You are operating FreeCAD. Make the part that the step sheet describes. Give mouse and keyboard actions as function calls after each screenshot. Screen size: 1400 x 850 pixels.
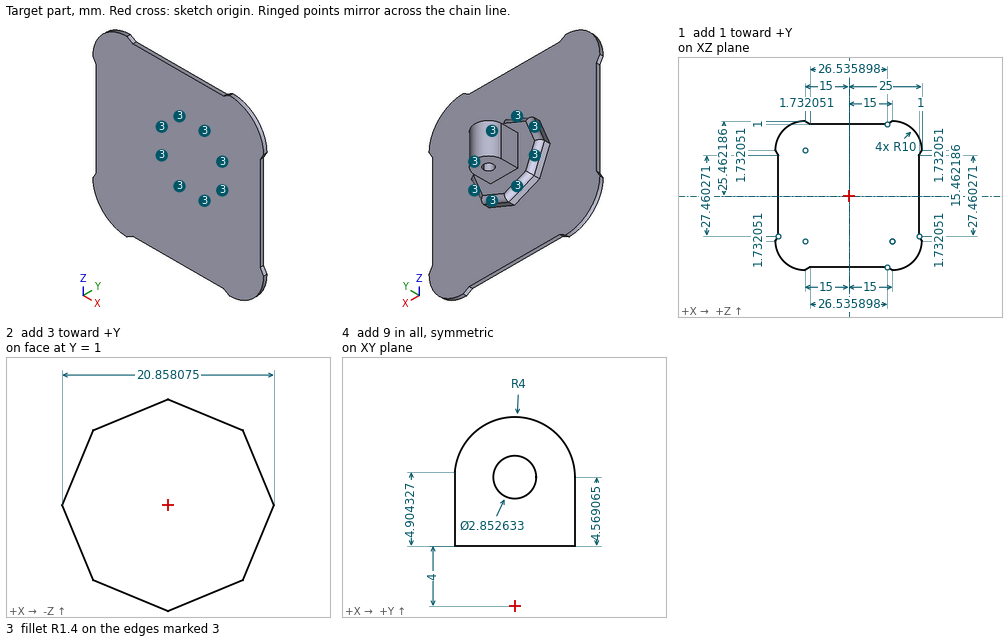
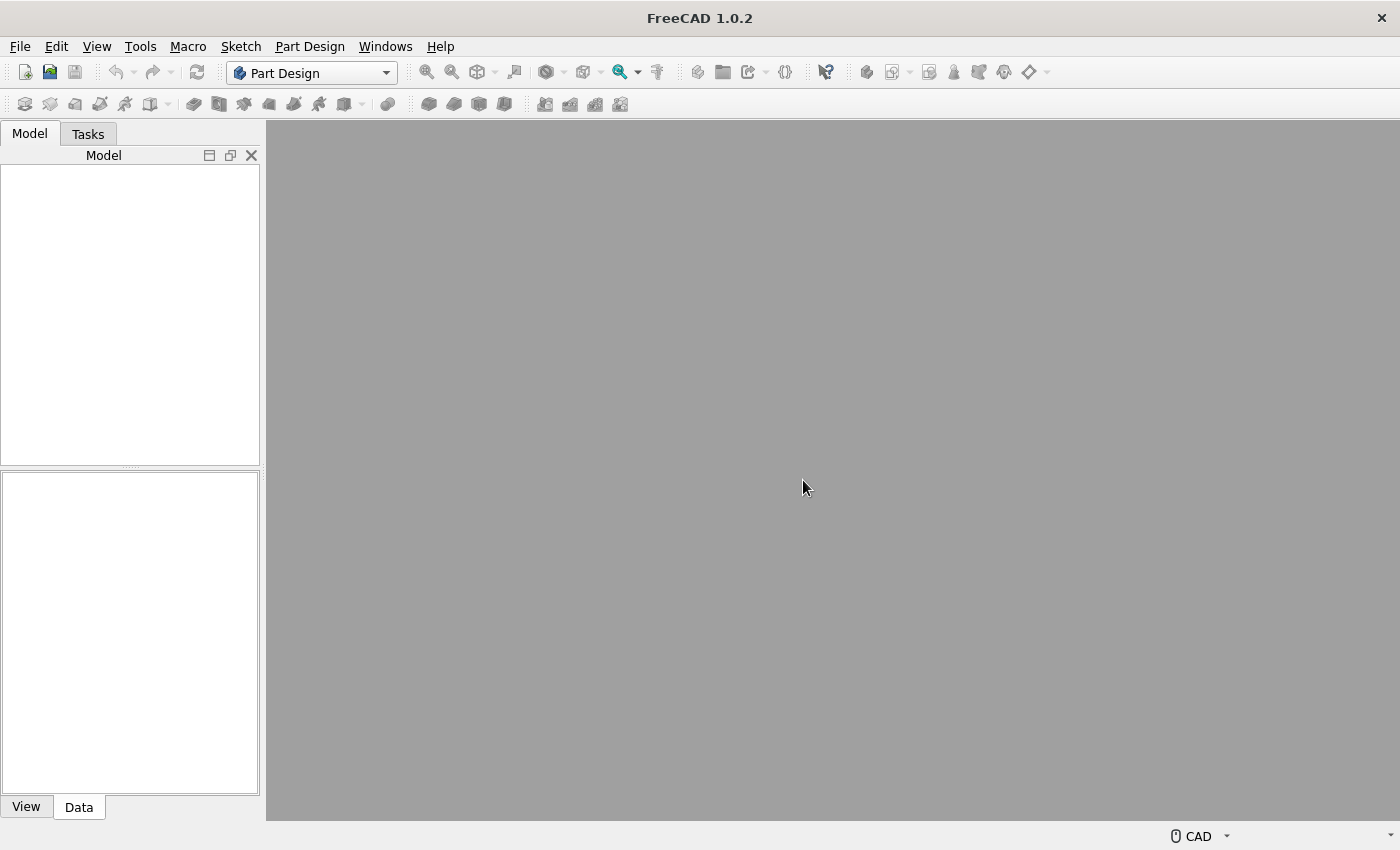
click(25, 72)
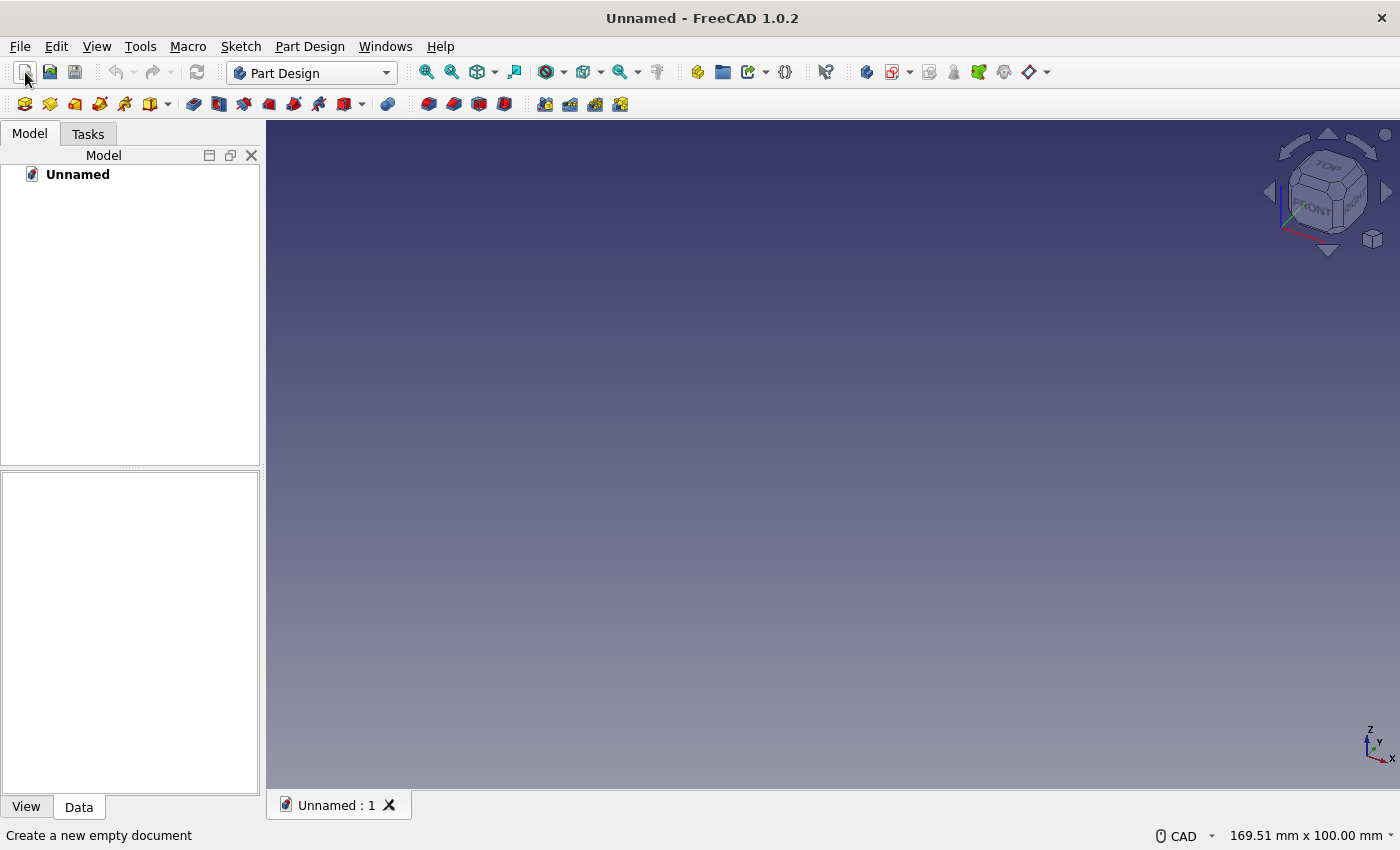
click(892, 72)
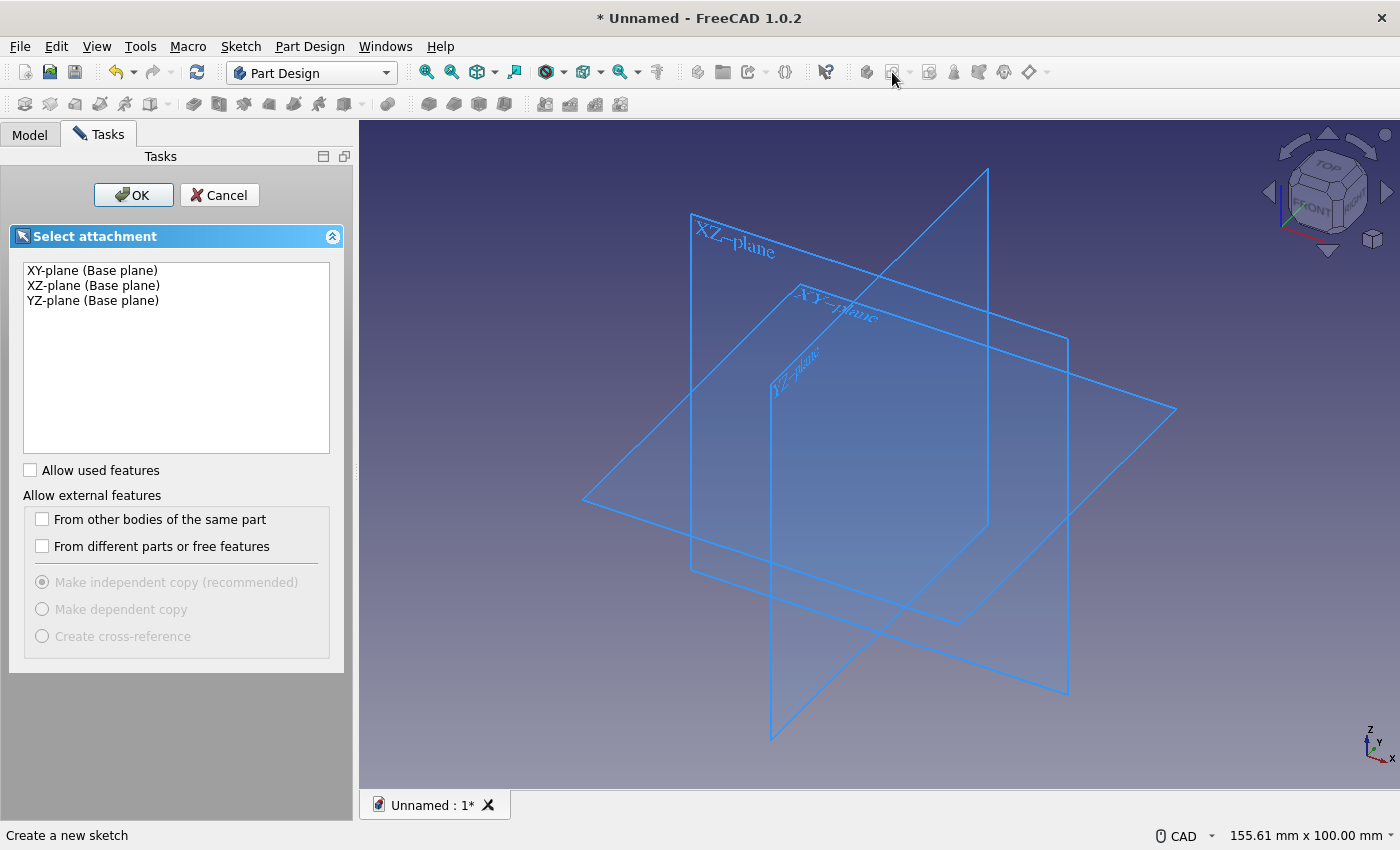
click(84, 286)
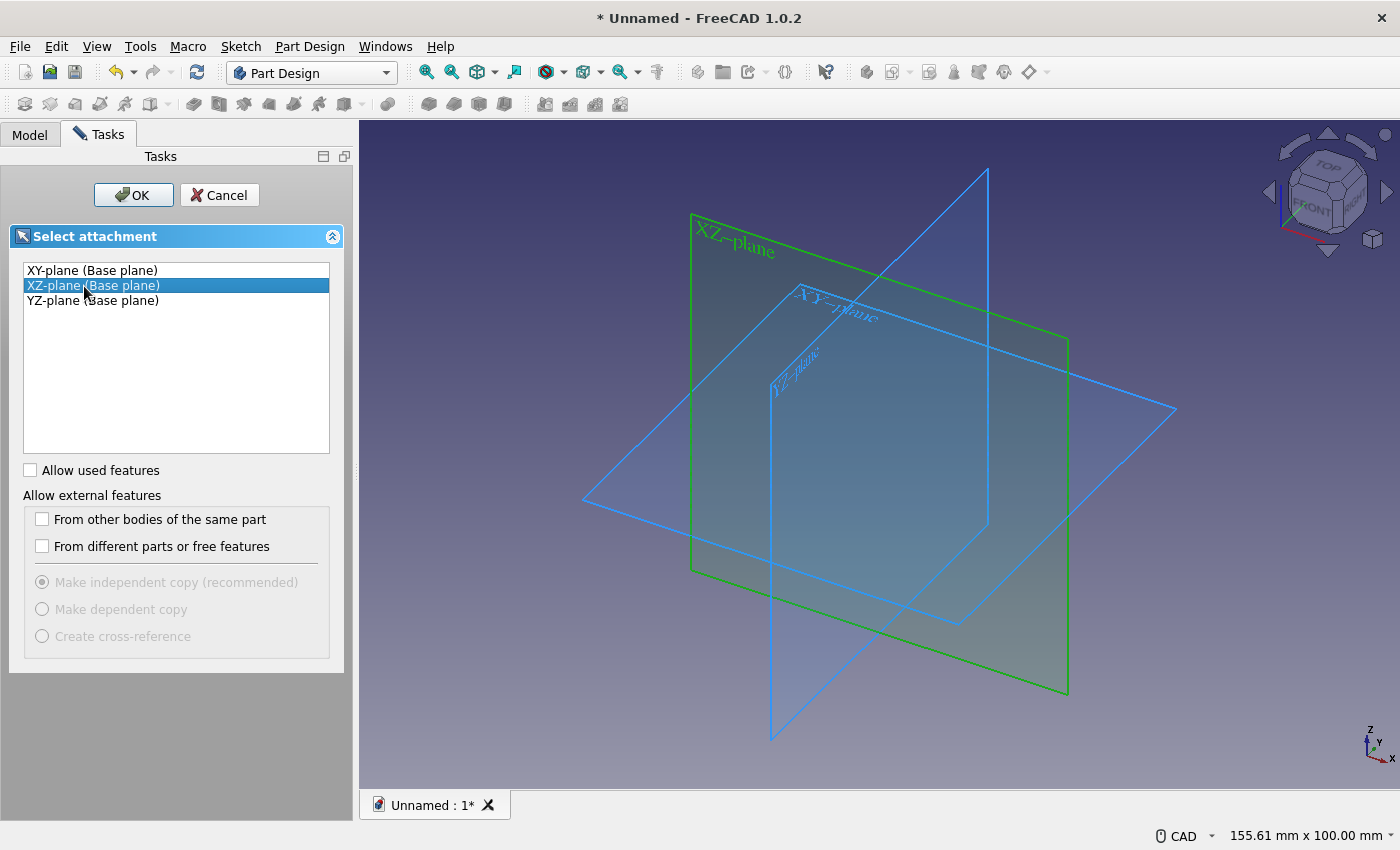
click(134, 195)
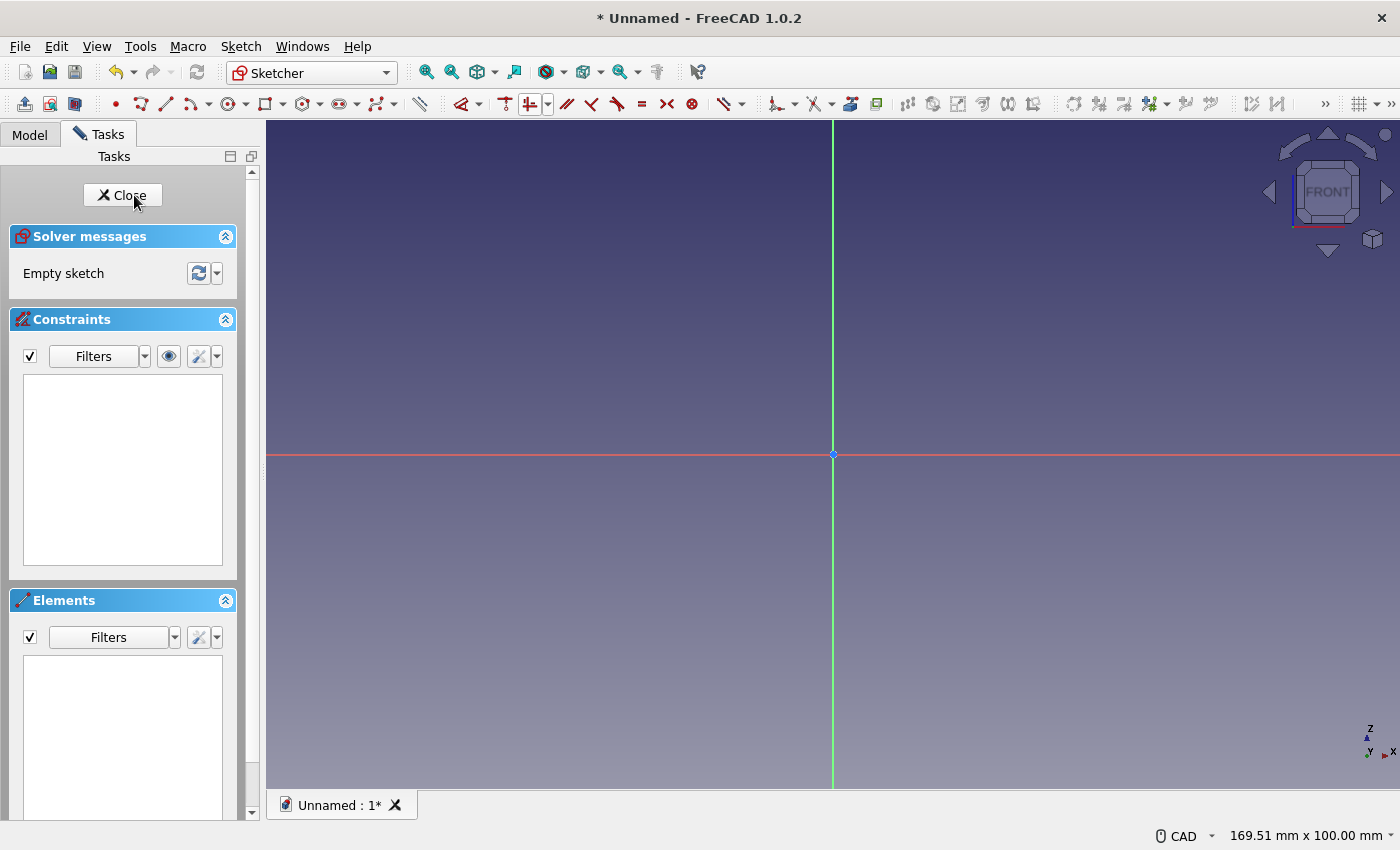
click(141, 104)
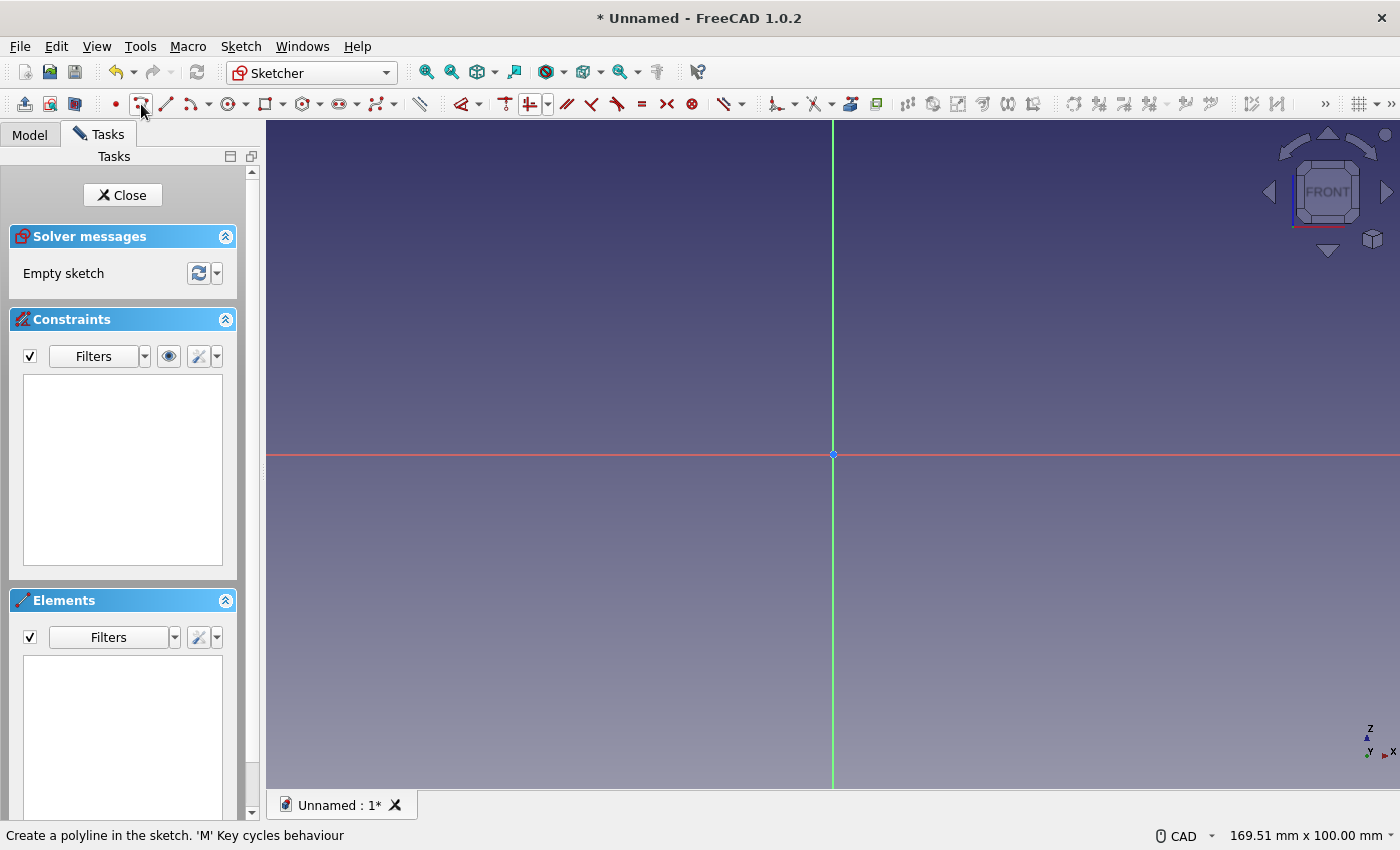
click(733, 284)
click(744, 291)
click(922, 291)
click(933, 284)
right_click(933, 284)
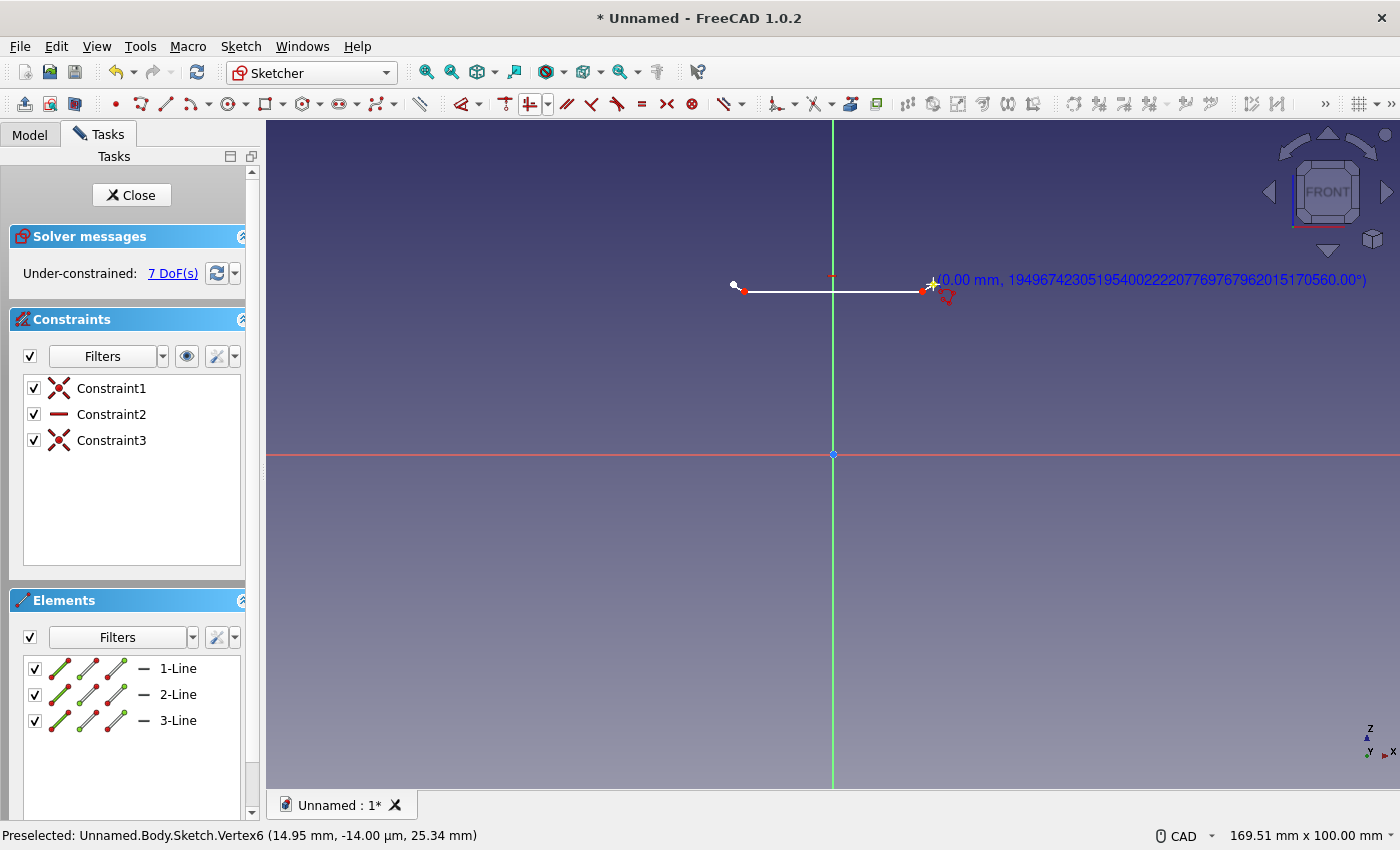
click(1000, 351)
click(994, 363)
click(994, 546)
click(1000, 558)
right_click(1000, 558)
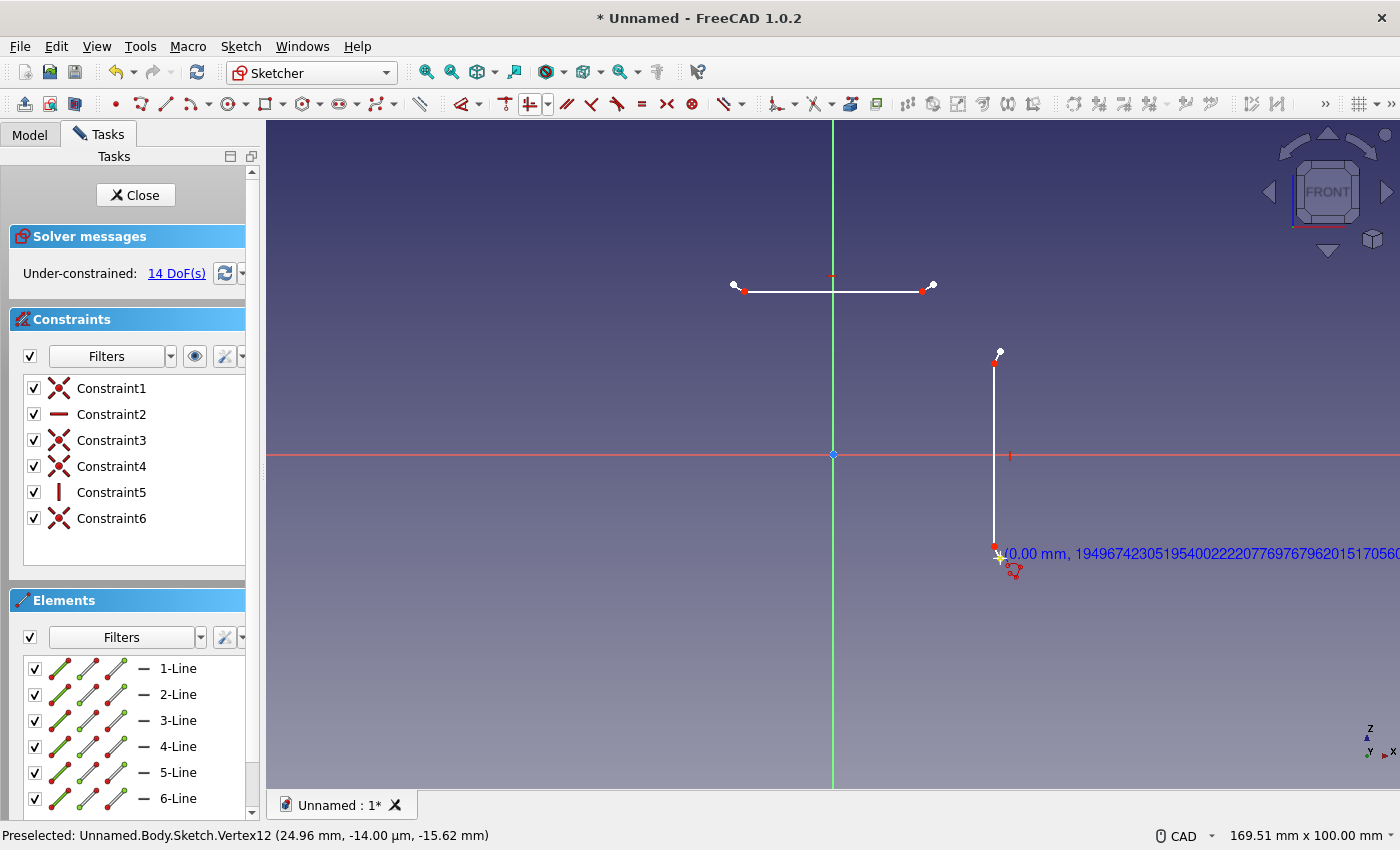
click(933, 625)
click(922, 618)
click(744, 618)
click(733, 625)
right_click(733, 625)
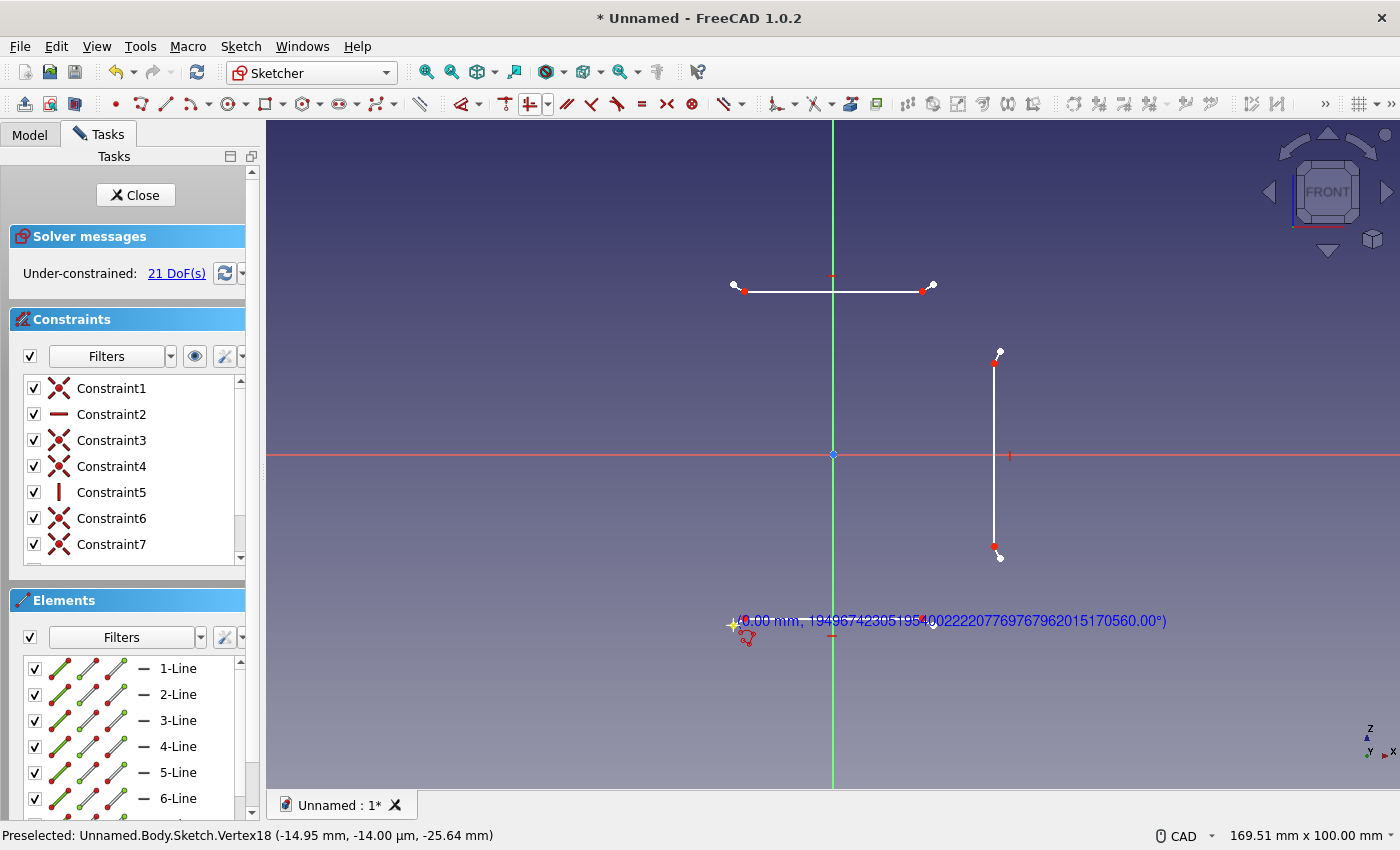
click(666, 558)
click(672, 546)
click(672, 363)
click(666, 351)
right_click(666, 351)